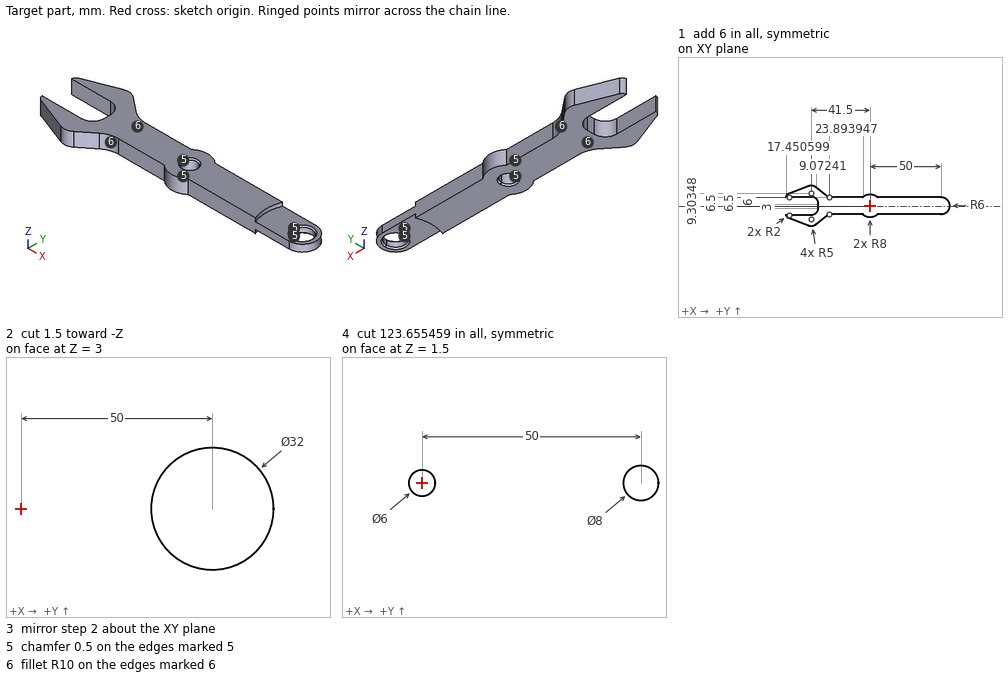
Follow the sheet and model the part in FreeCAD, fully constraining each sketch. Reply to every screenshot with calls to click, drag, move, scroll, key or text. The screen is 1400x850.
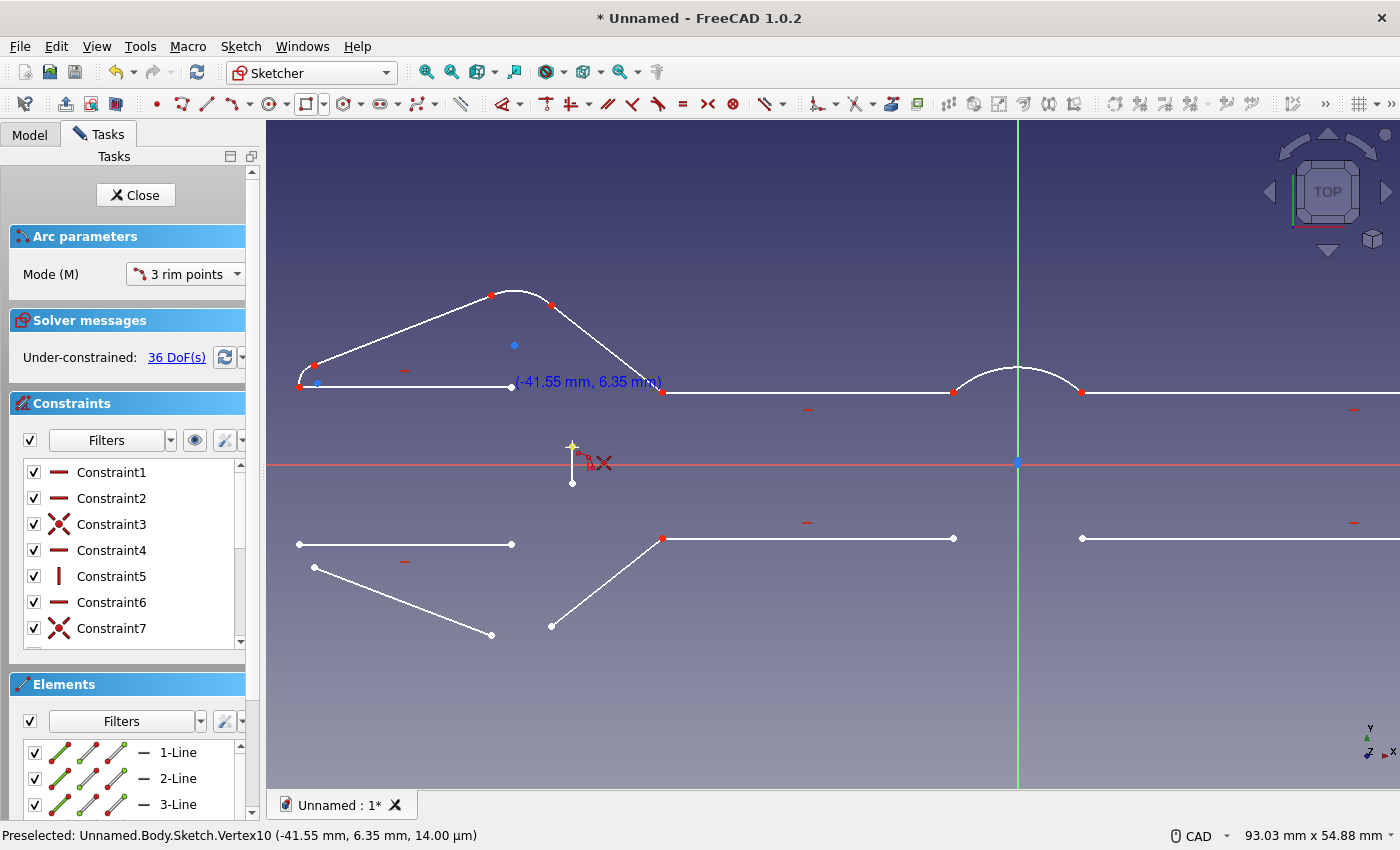
click(572, 447)
click(555, 403)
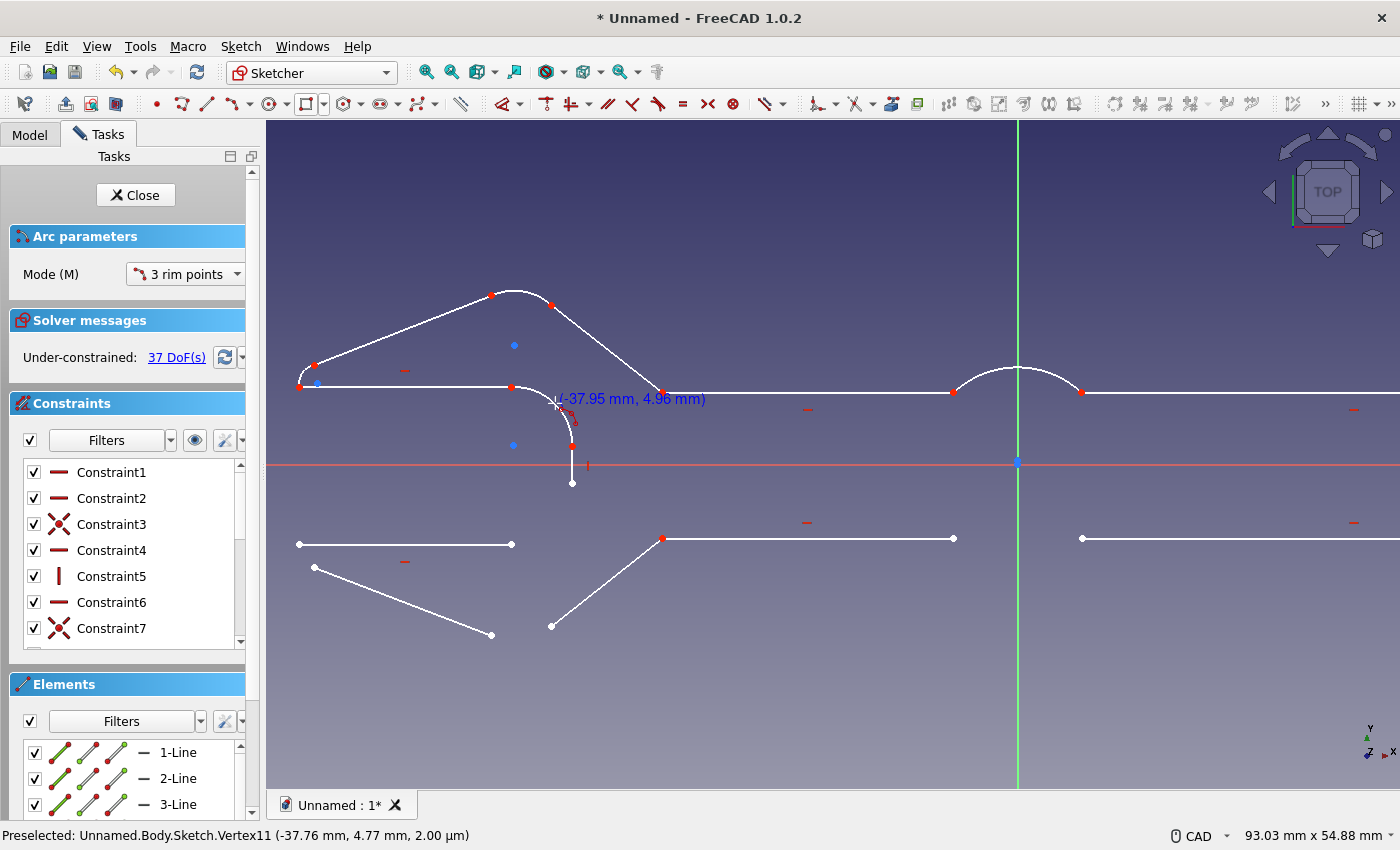
click(572, 484)
click(511, 545)
click(555, 526)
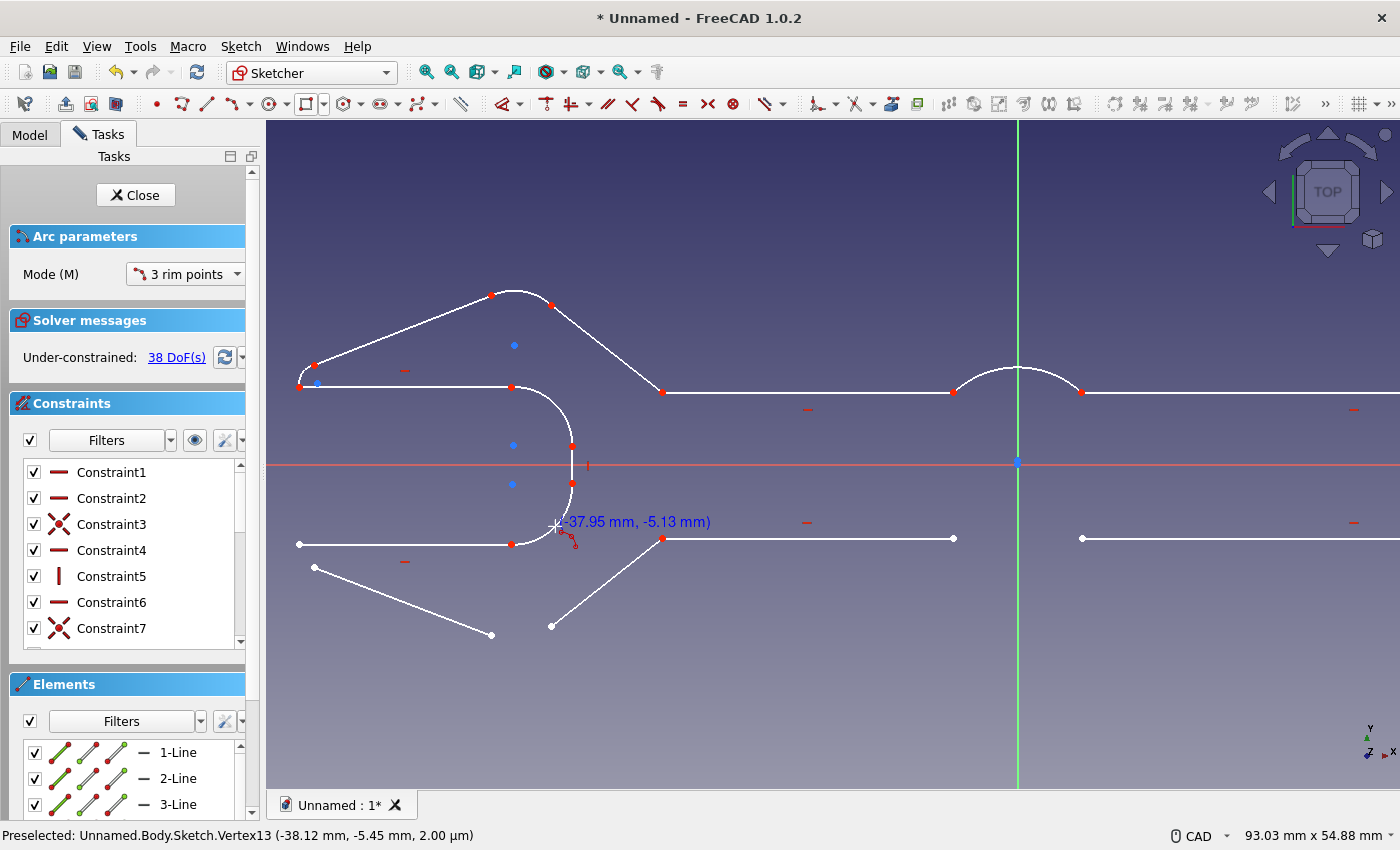
click(299, 545)
click(314, 568)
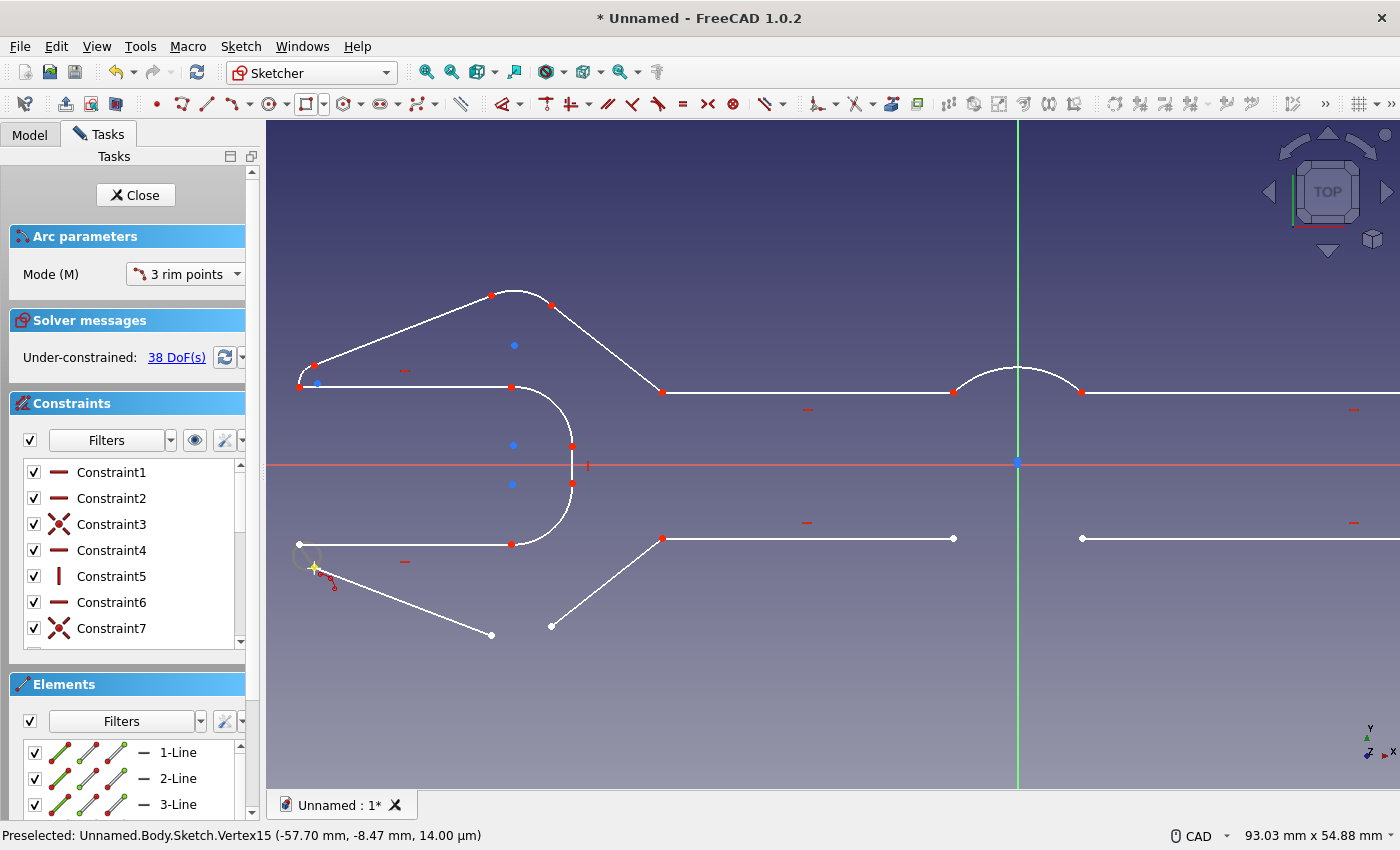
scroll(303, 558, up, 7)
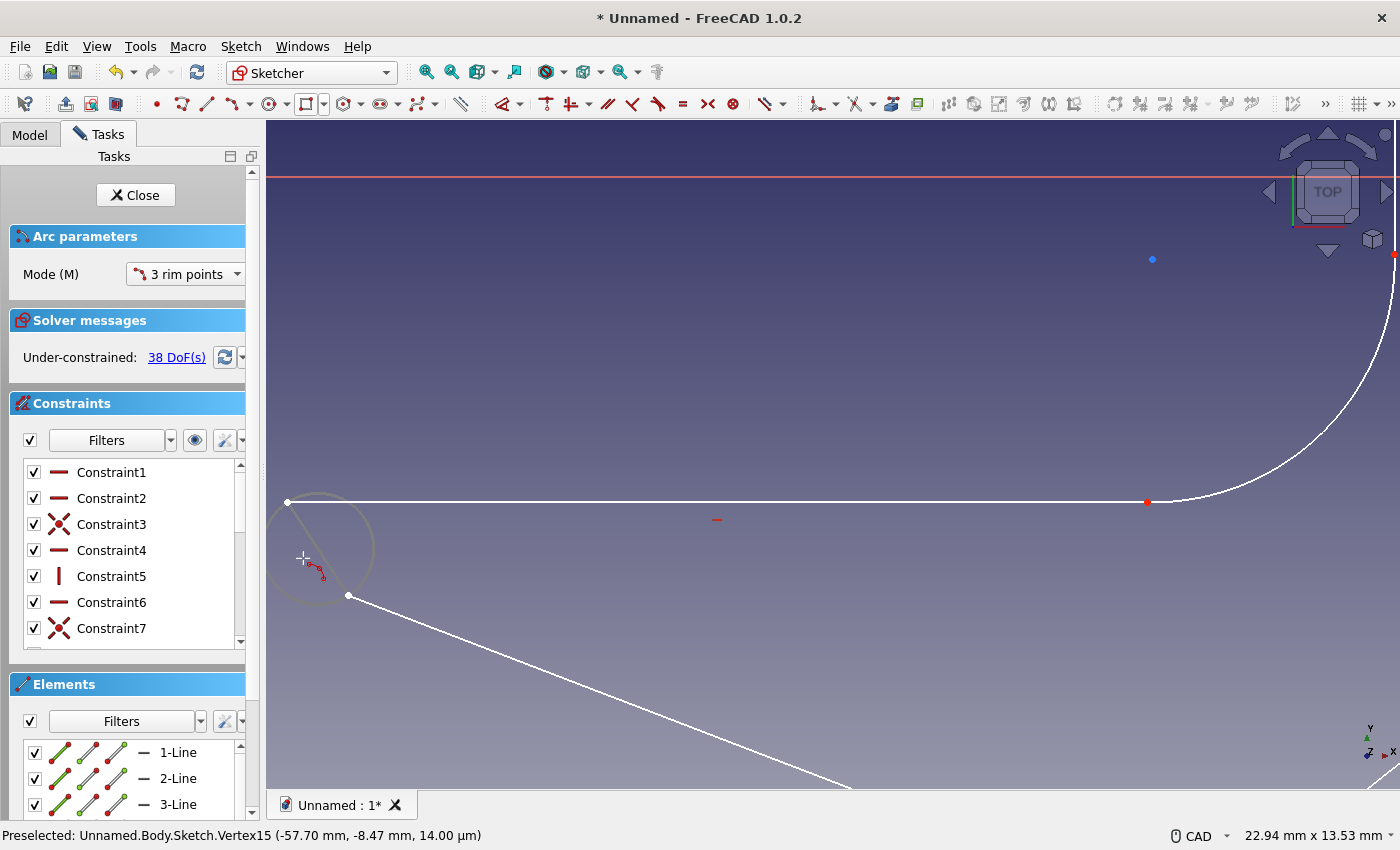
click(304, 554)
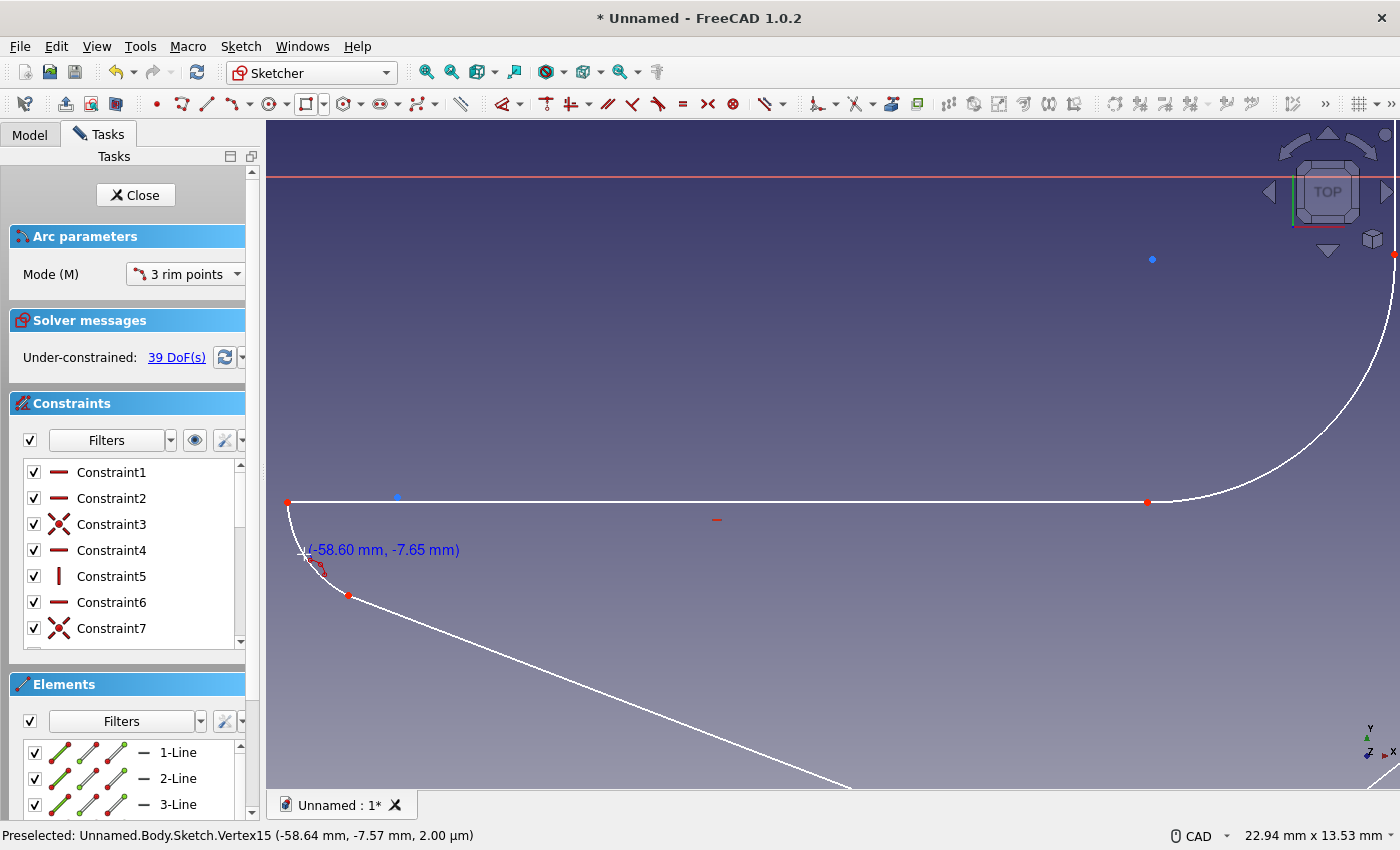
scroll(470, 489, down, 11)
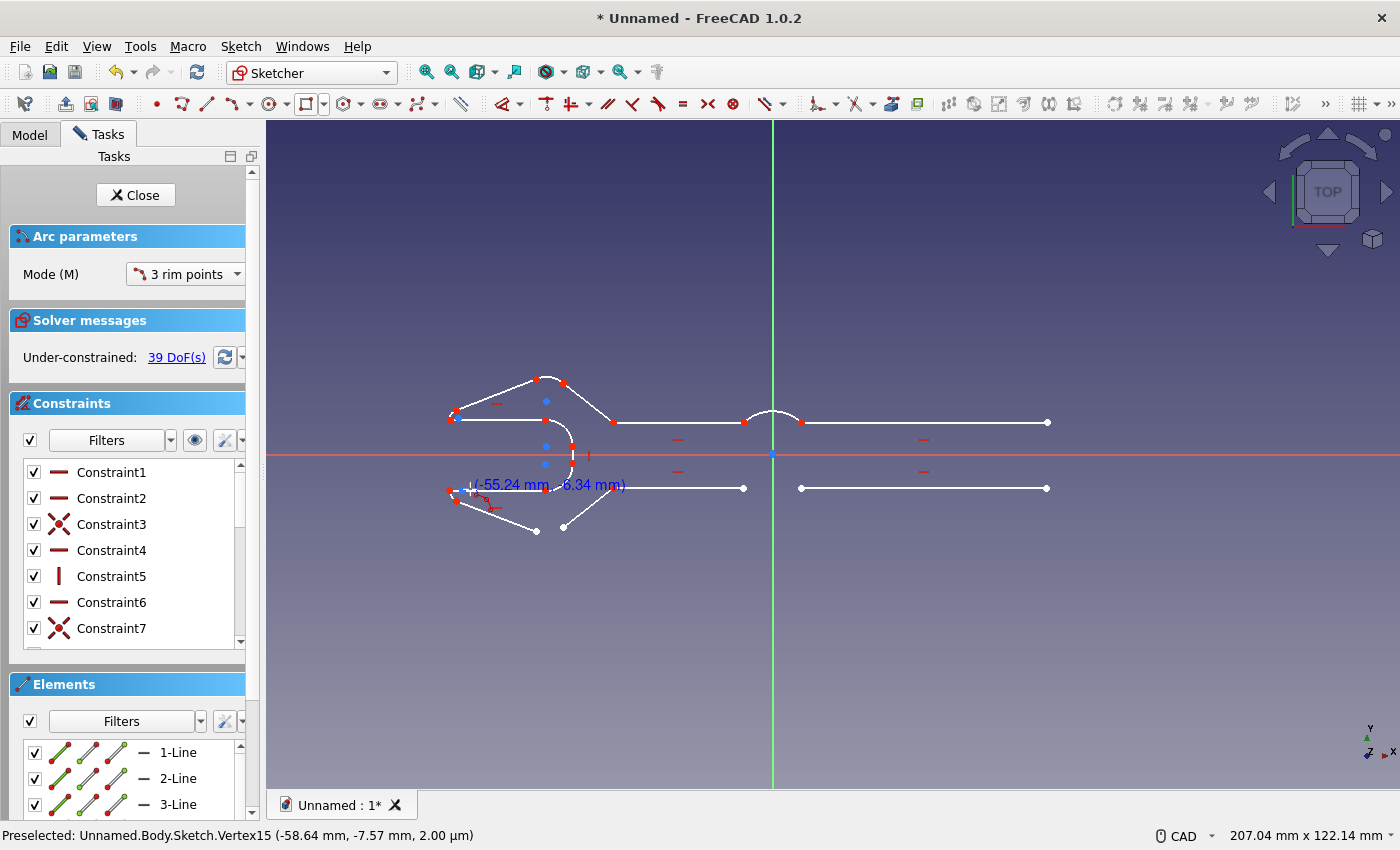
click(536, 532)
click(563, 528)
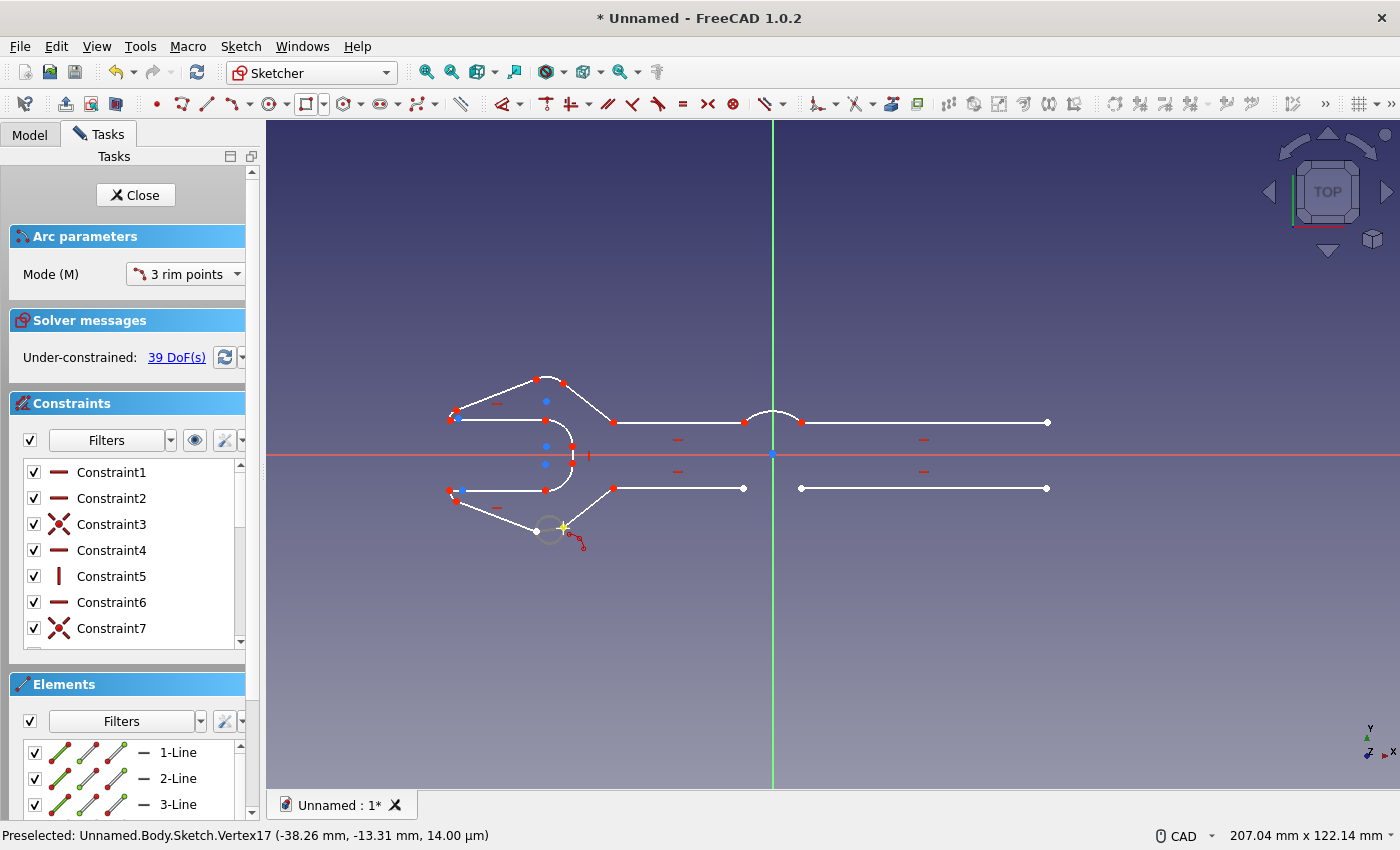
scroll(550, 533, up, 8)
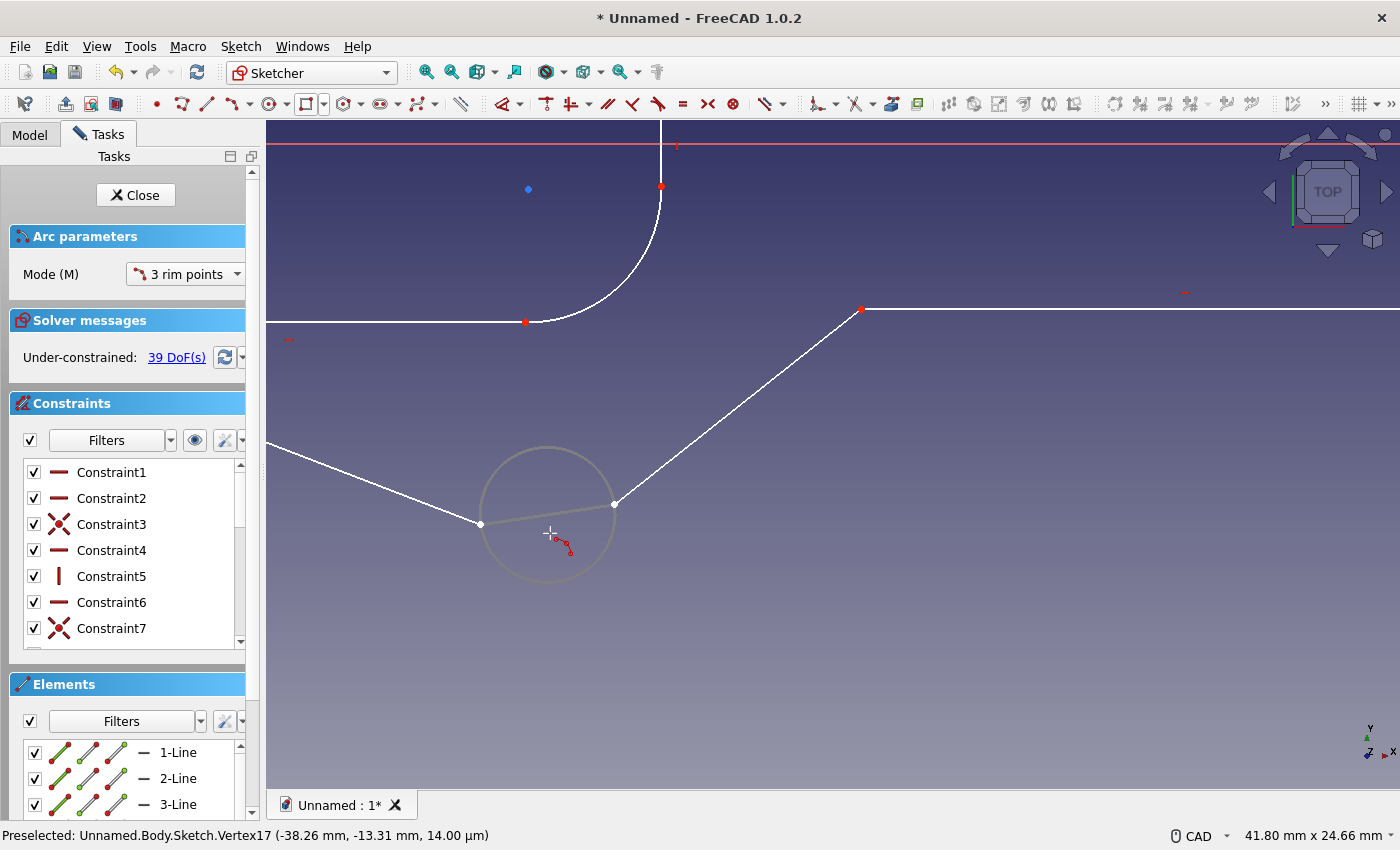
click(550, 530)